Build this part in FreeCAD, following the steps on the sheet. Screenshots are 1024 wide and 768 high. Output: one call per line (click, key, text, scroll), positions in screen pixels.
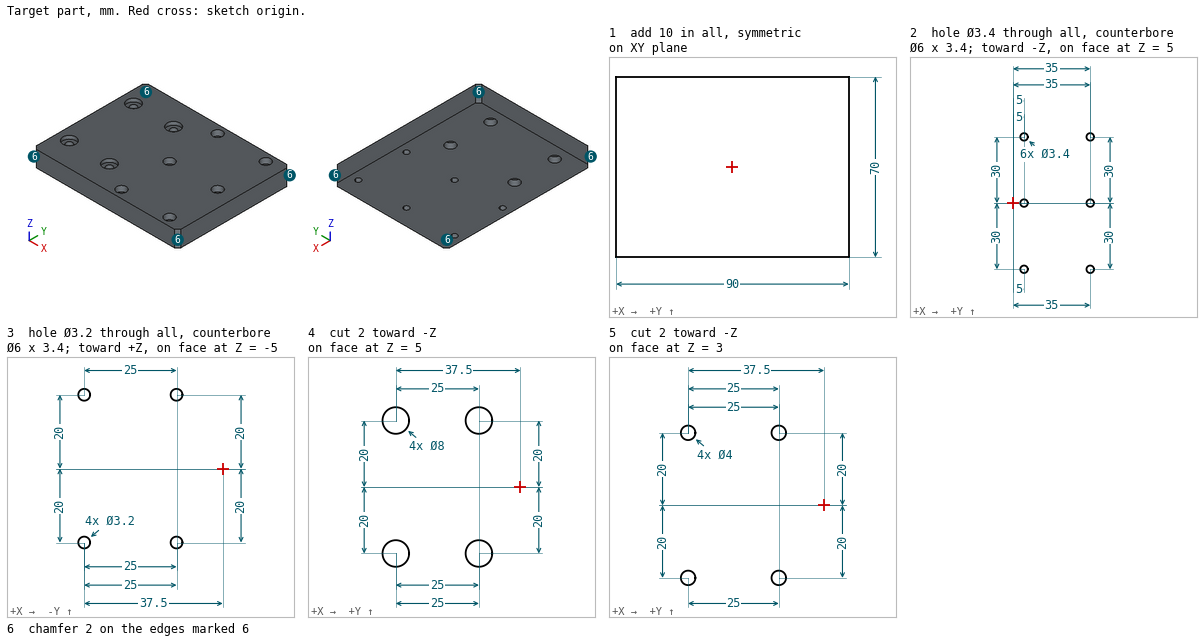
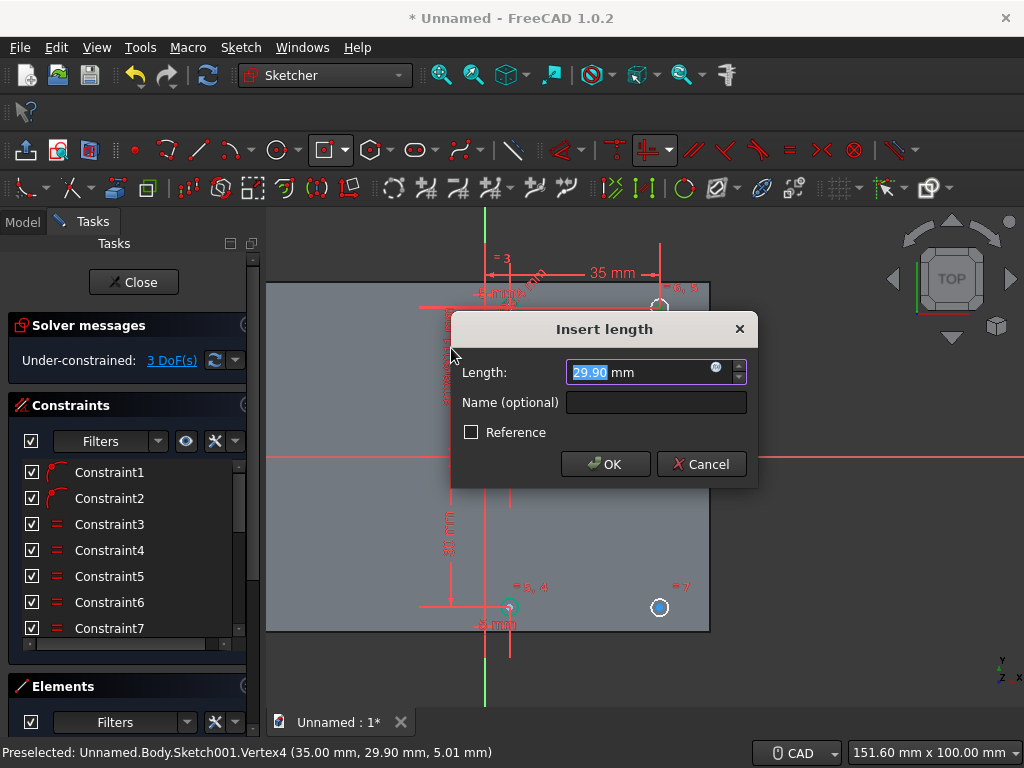
text(30)
key(Return)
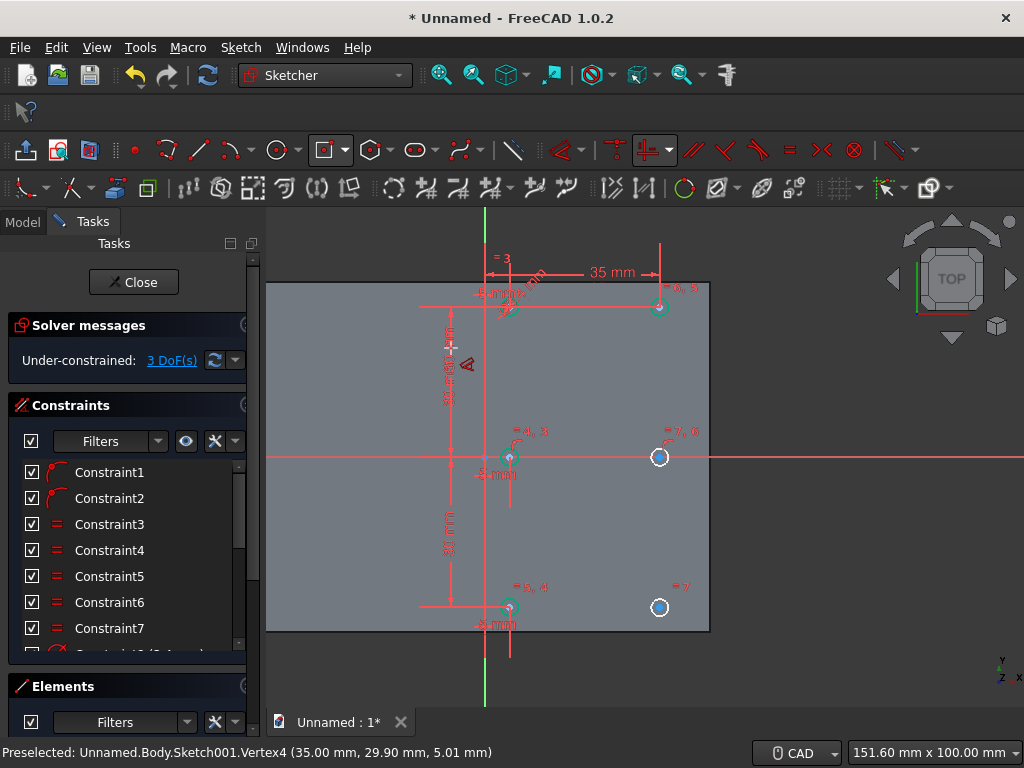
click(660, 457)
click(572, 491)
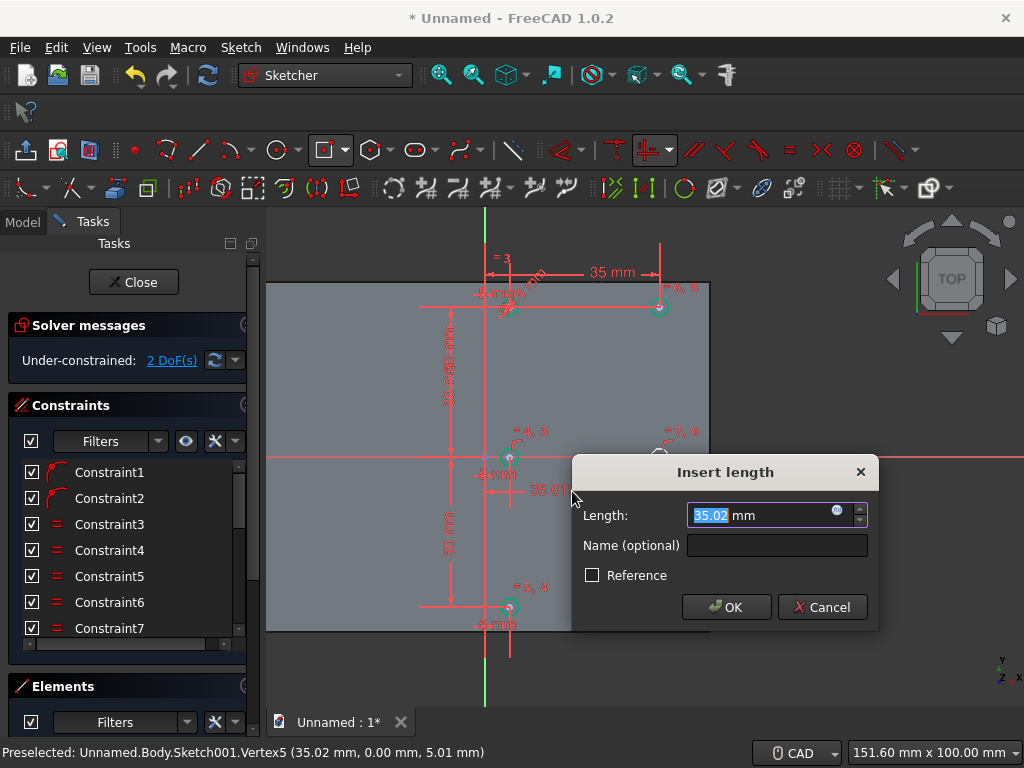
text(35)
key(Return)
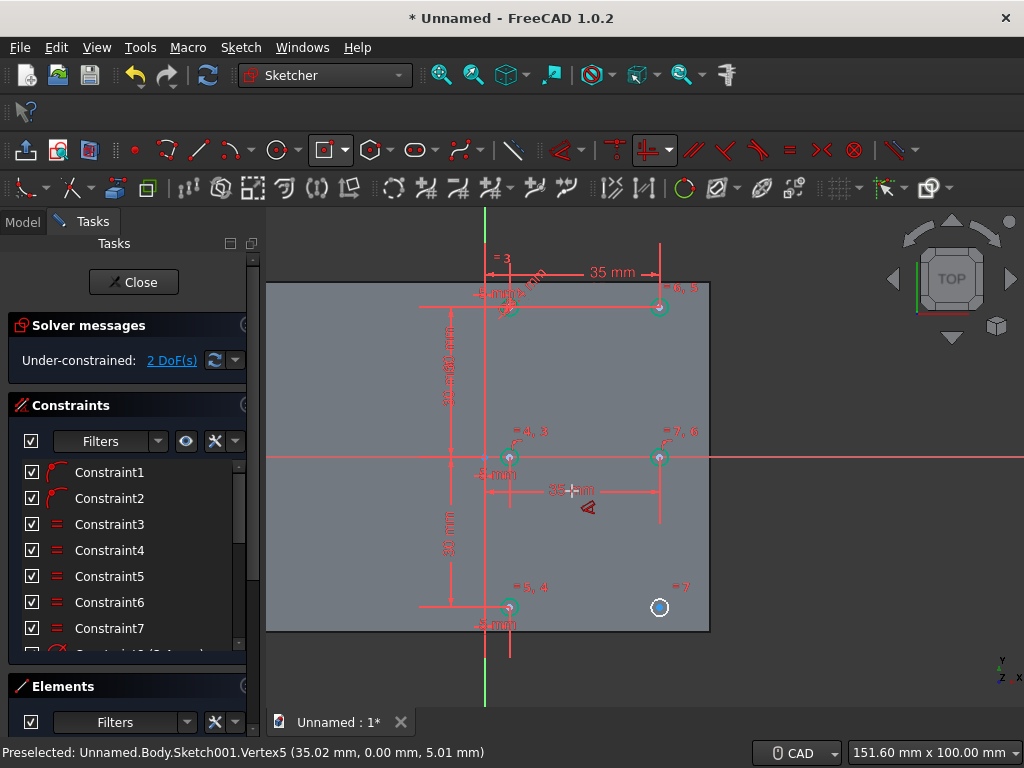
click(660, 608)
click(572, 642)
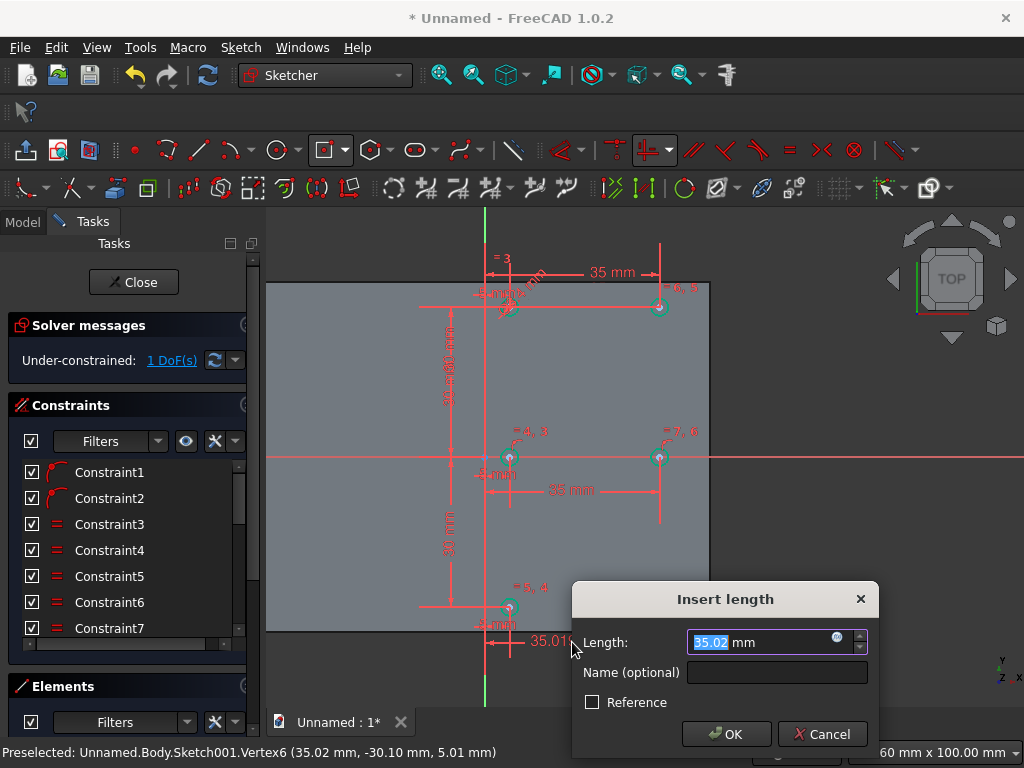
text(35)
key(Return)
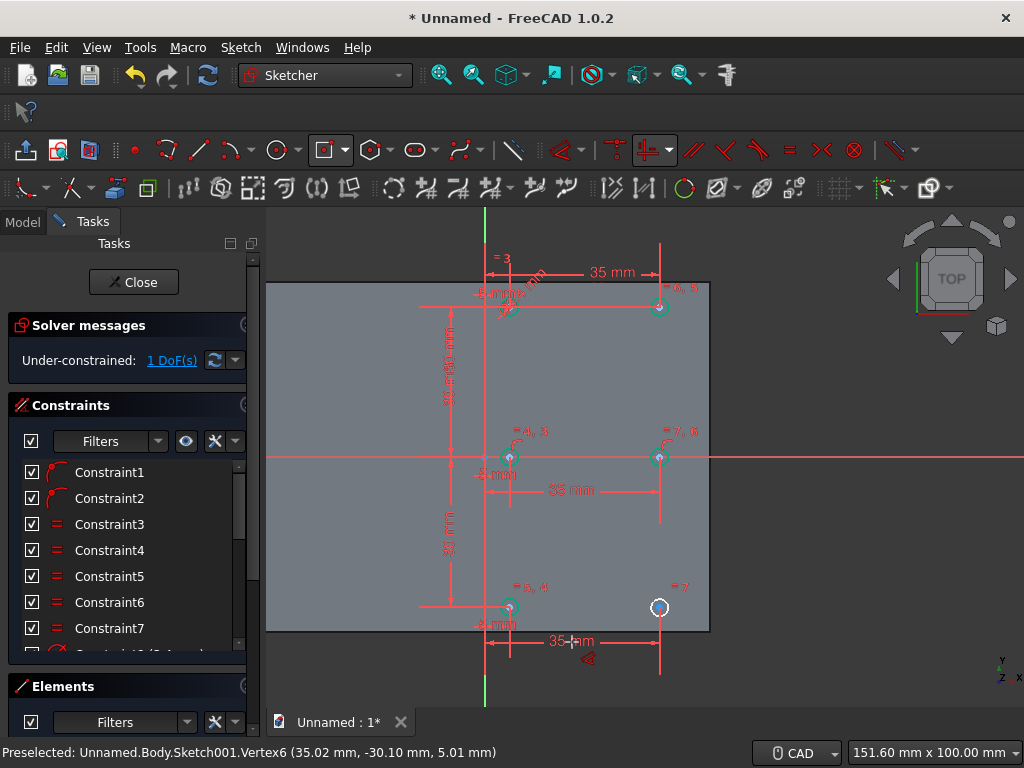
click(660, 608)
click(451, 498)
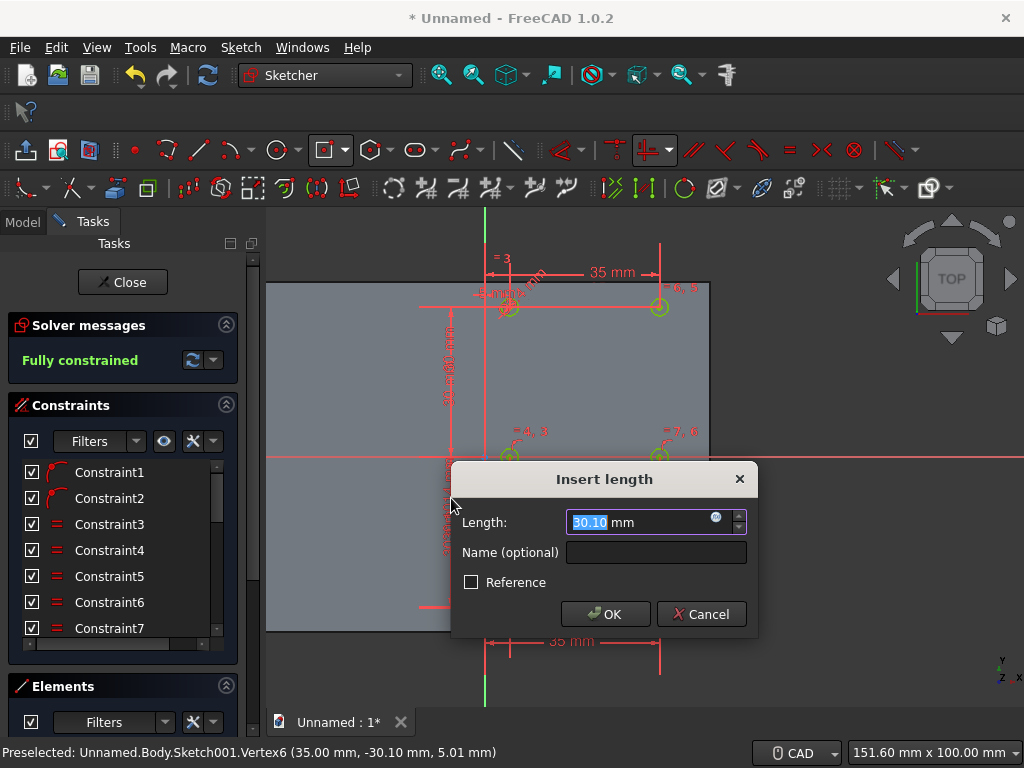
text(30)
key(Return)
key(Escape)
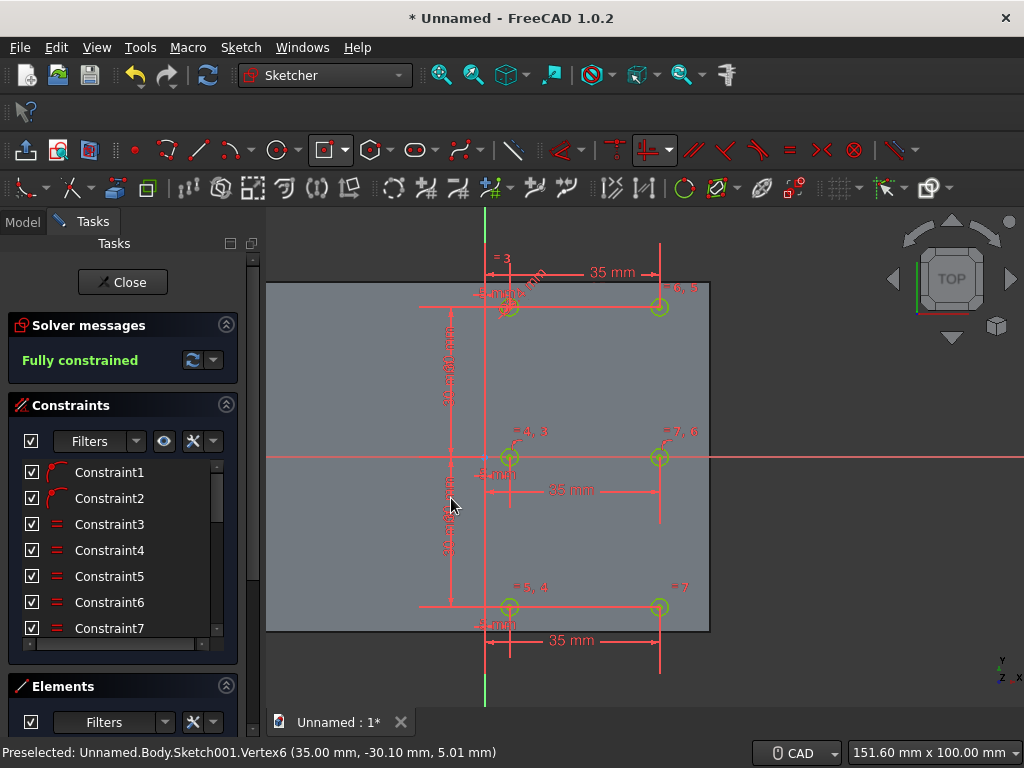
click(123, 282)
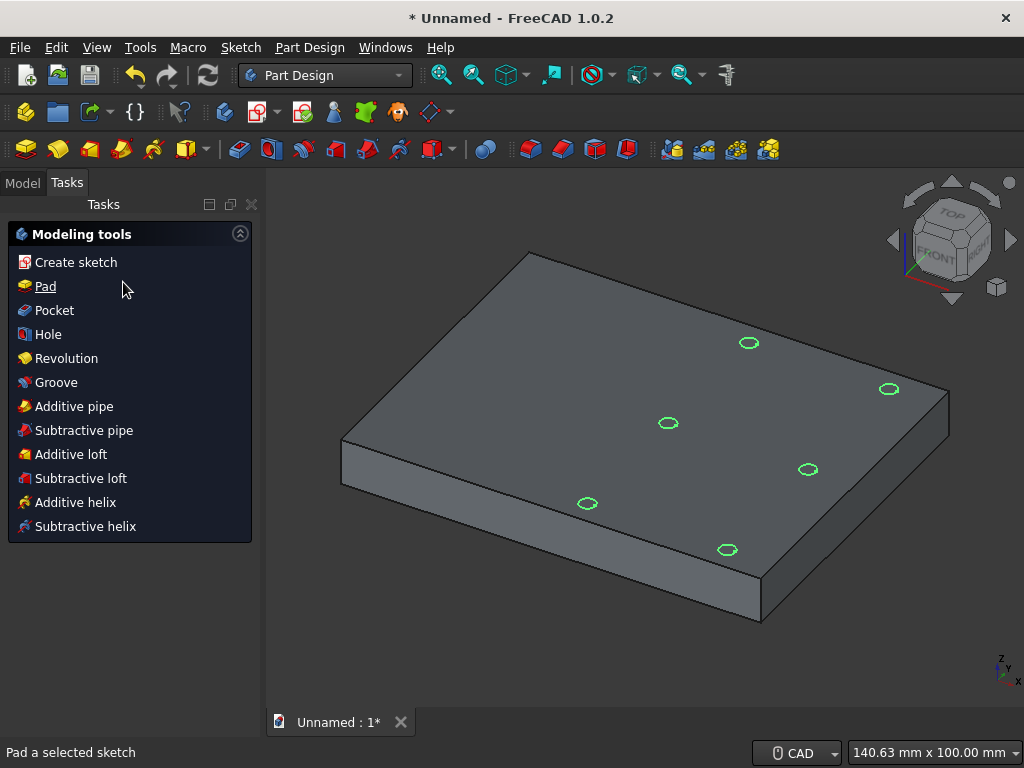
click(272, 150)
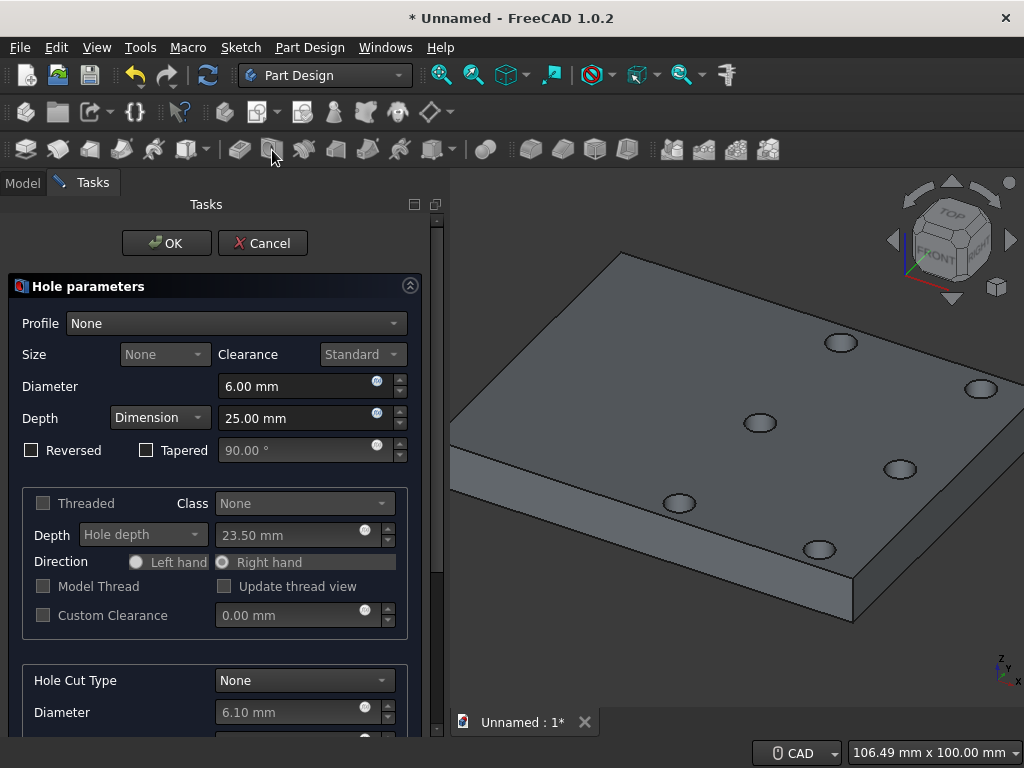
triple_click(305, 386)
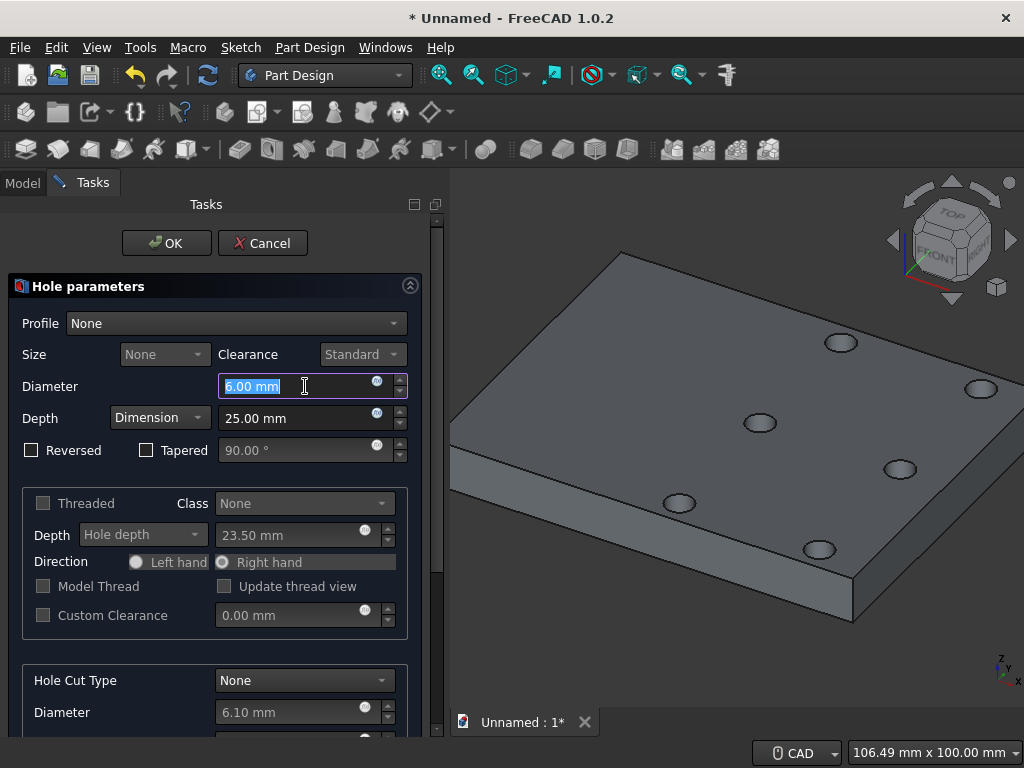
text(3.4)
key(Tab)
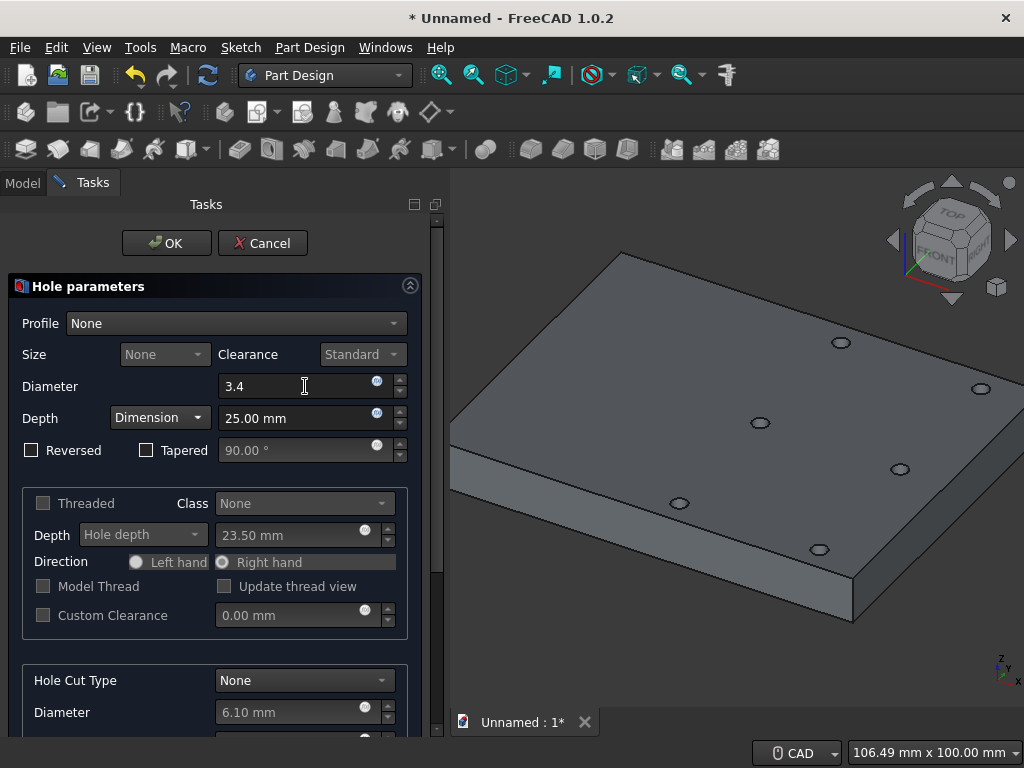
click(161, 418)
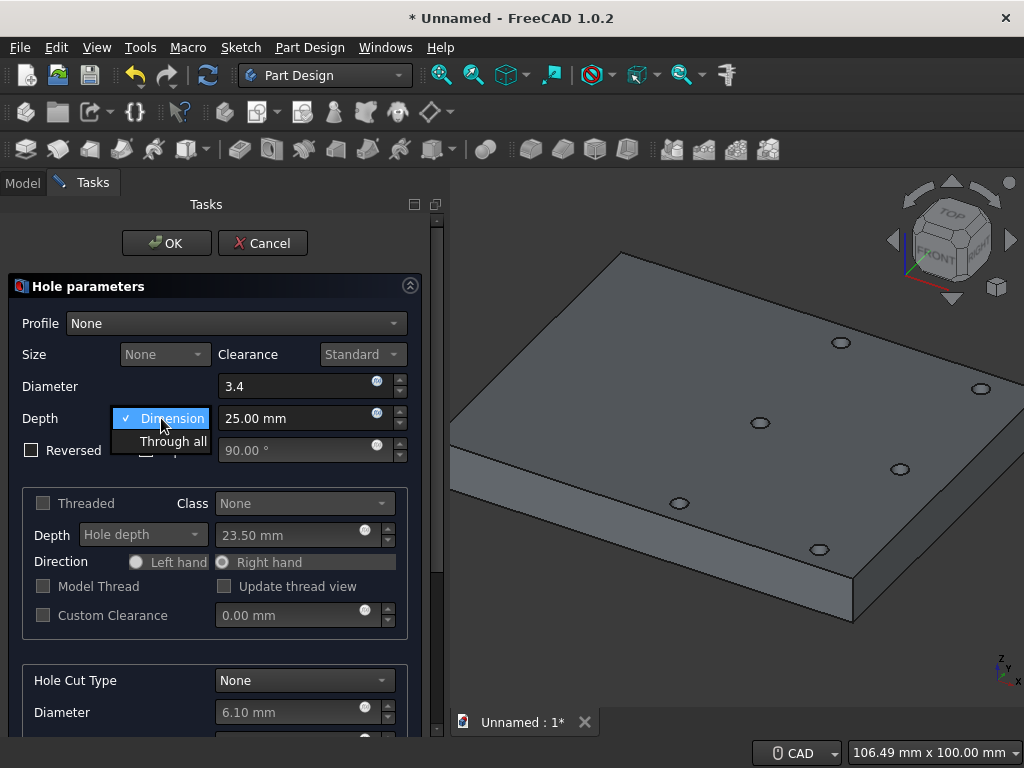
click(160, 442)